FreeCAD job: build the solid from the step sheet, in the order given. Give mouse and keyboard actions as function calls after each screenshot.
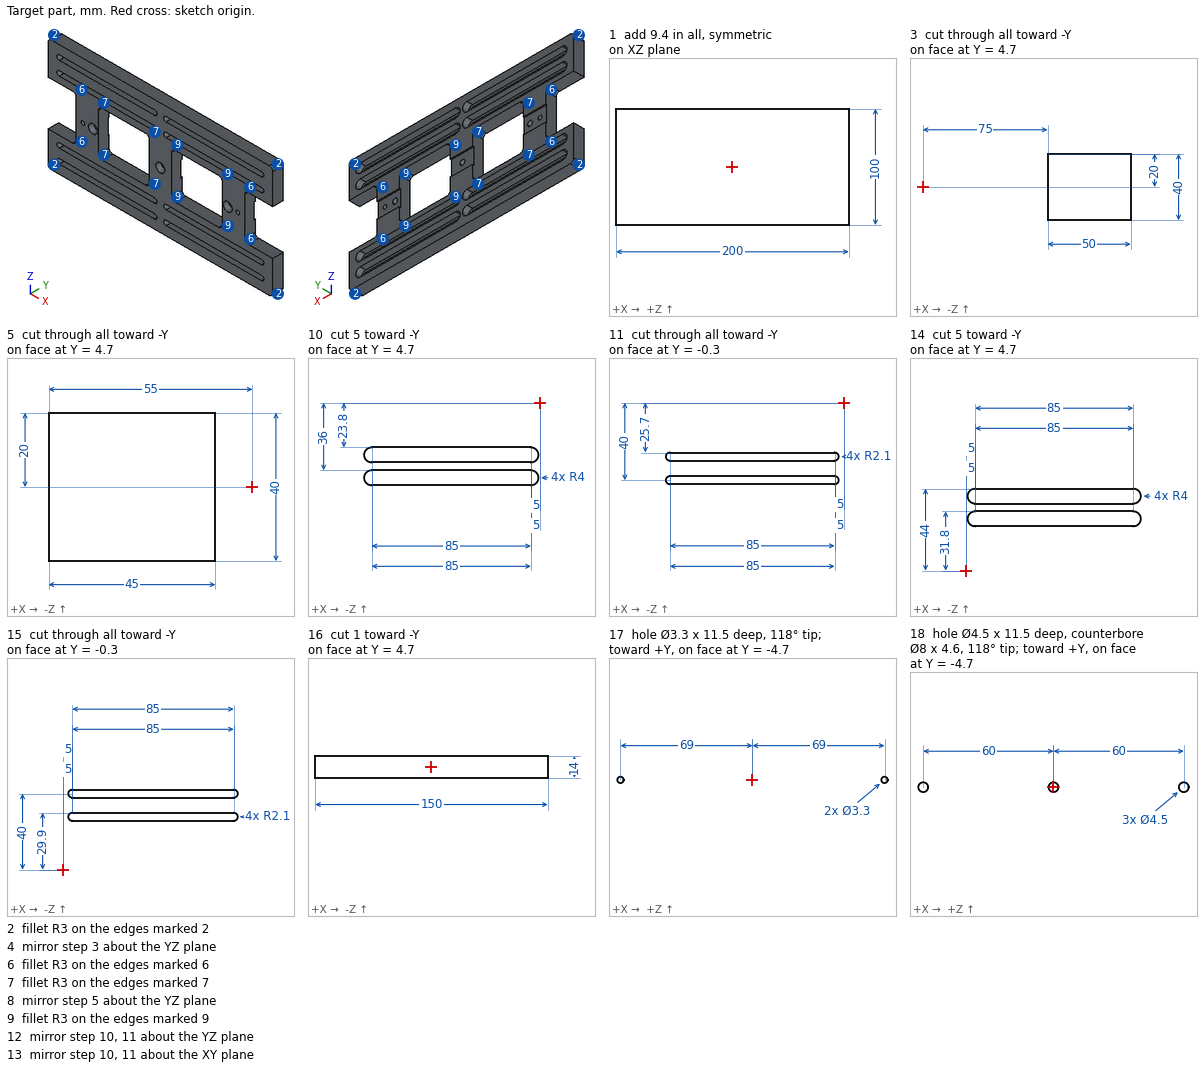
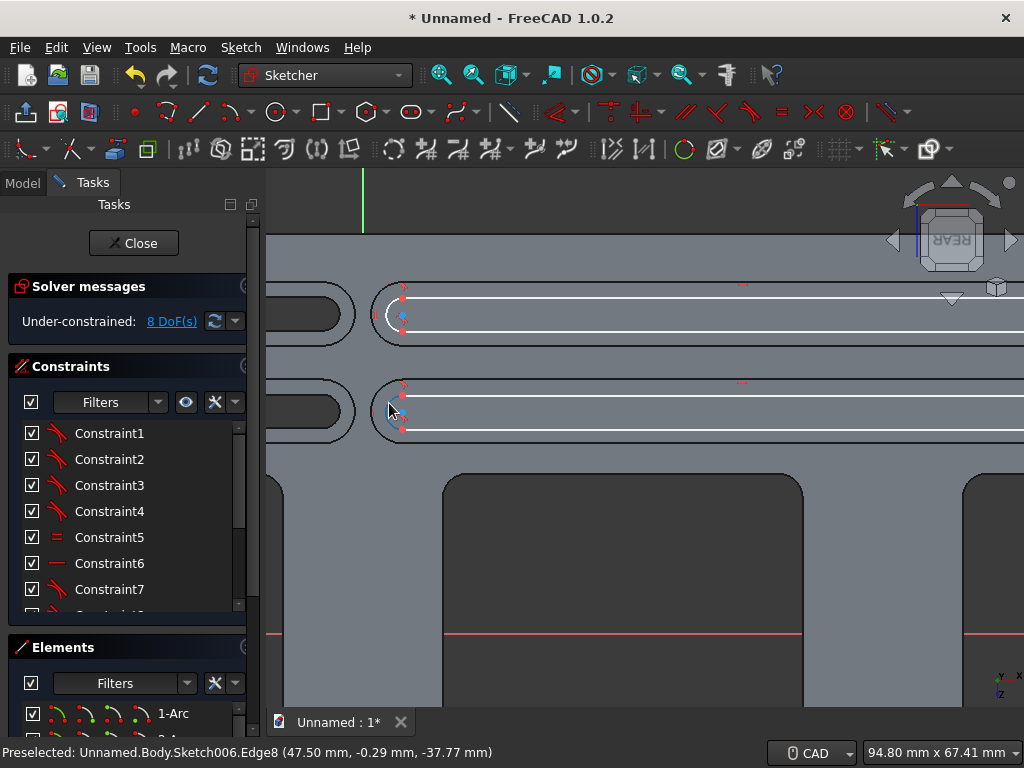
click(389, 403)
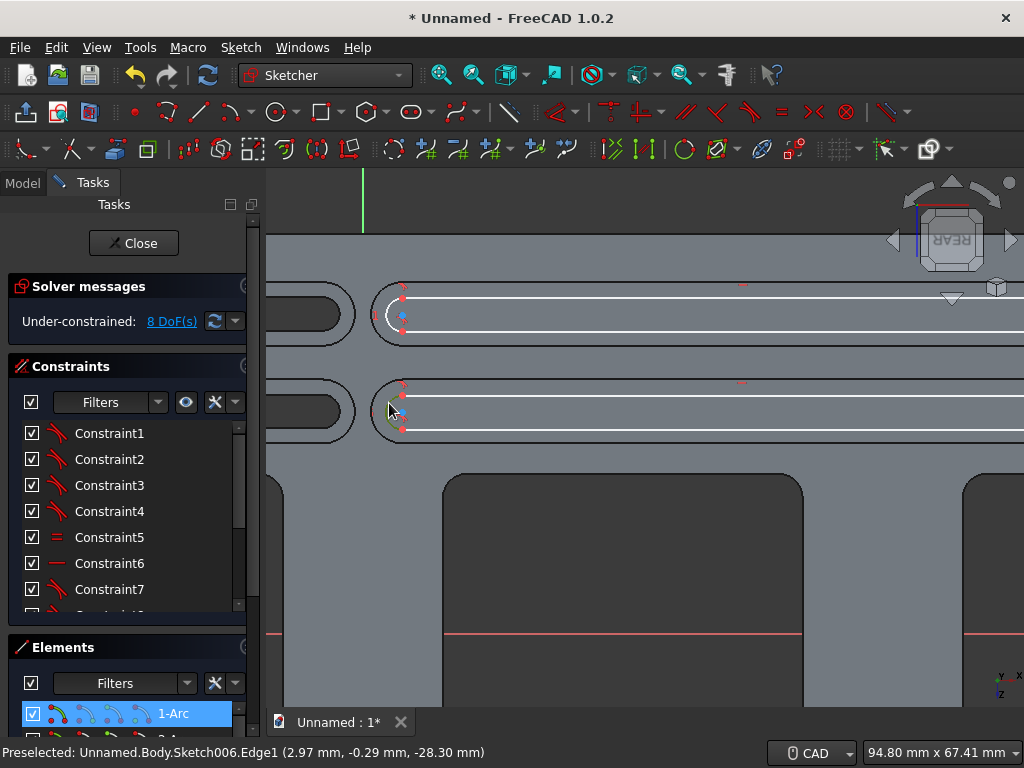
click(389, 305)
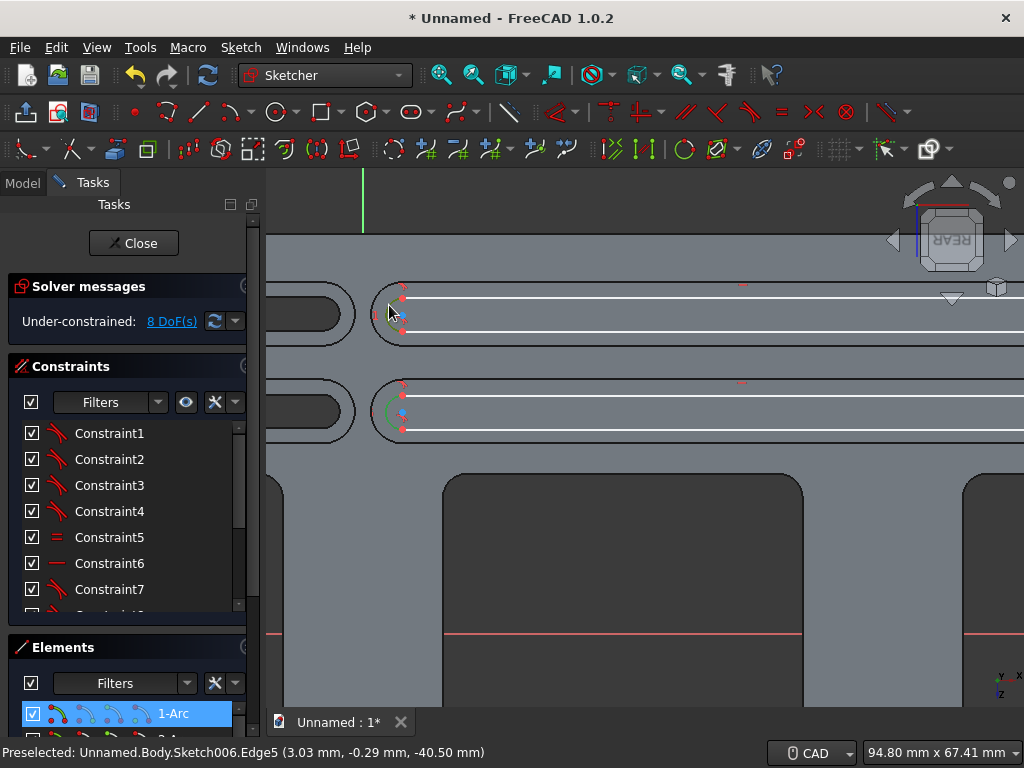
key(e)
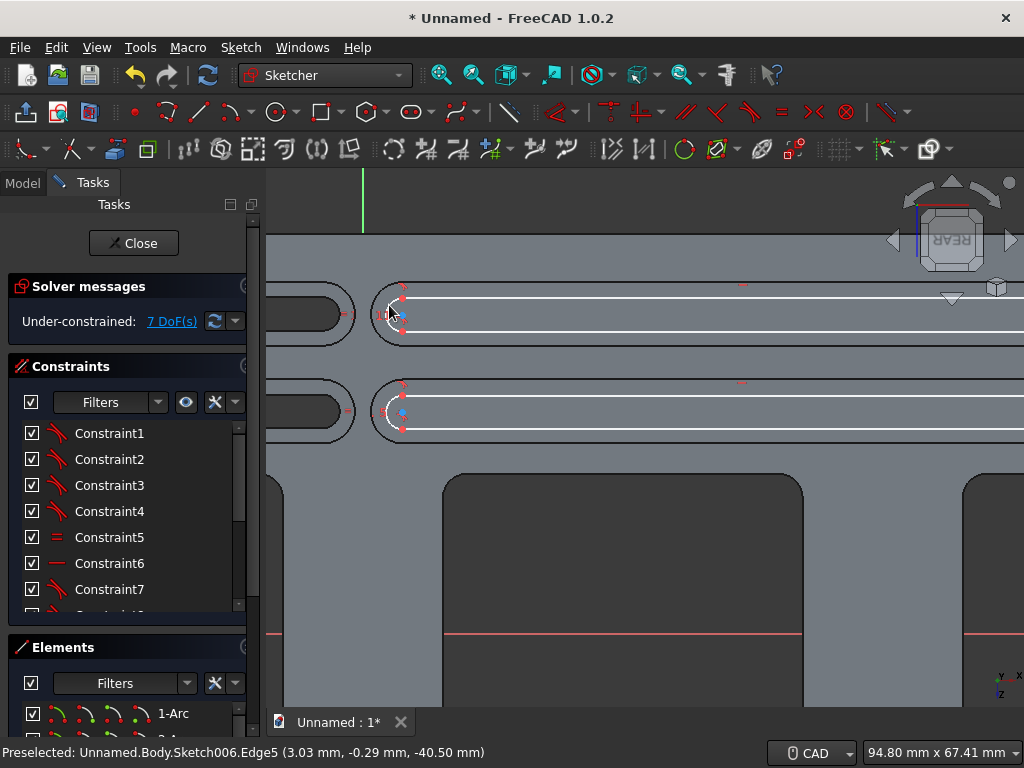
key(d)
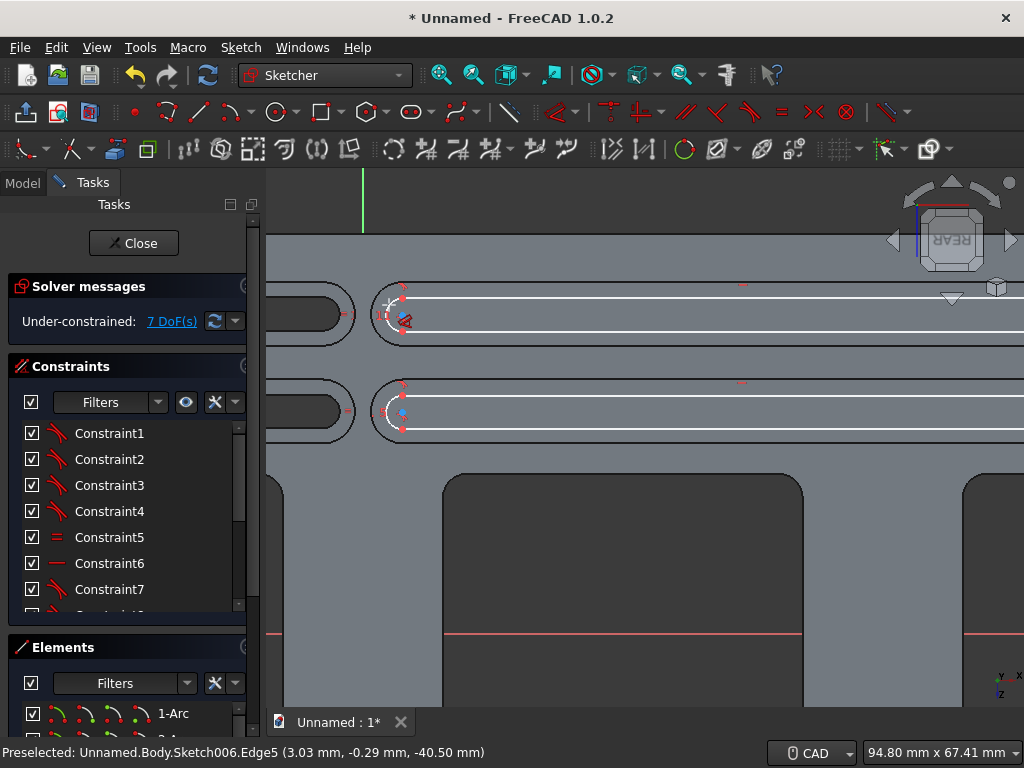
scroll(389, 403, up, 5)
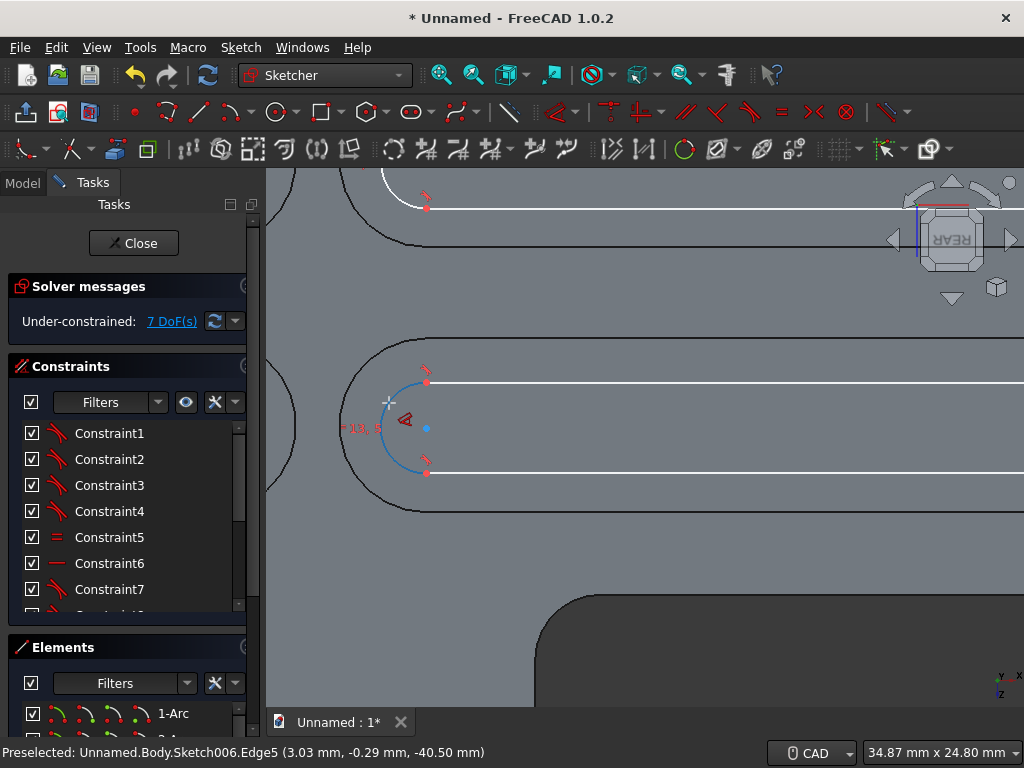
click(389, 401)
click(363, 382)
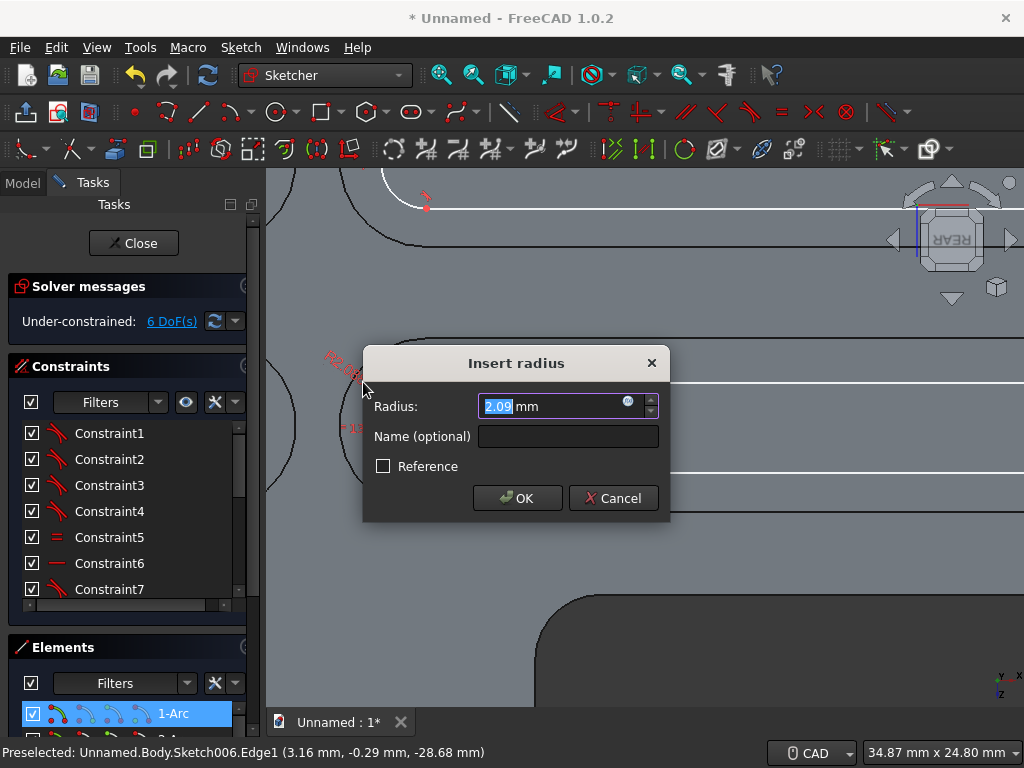
text(2.1)
key(Return)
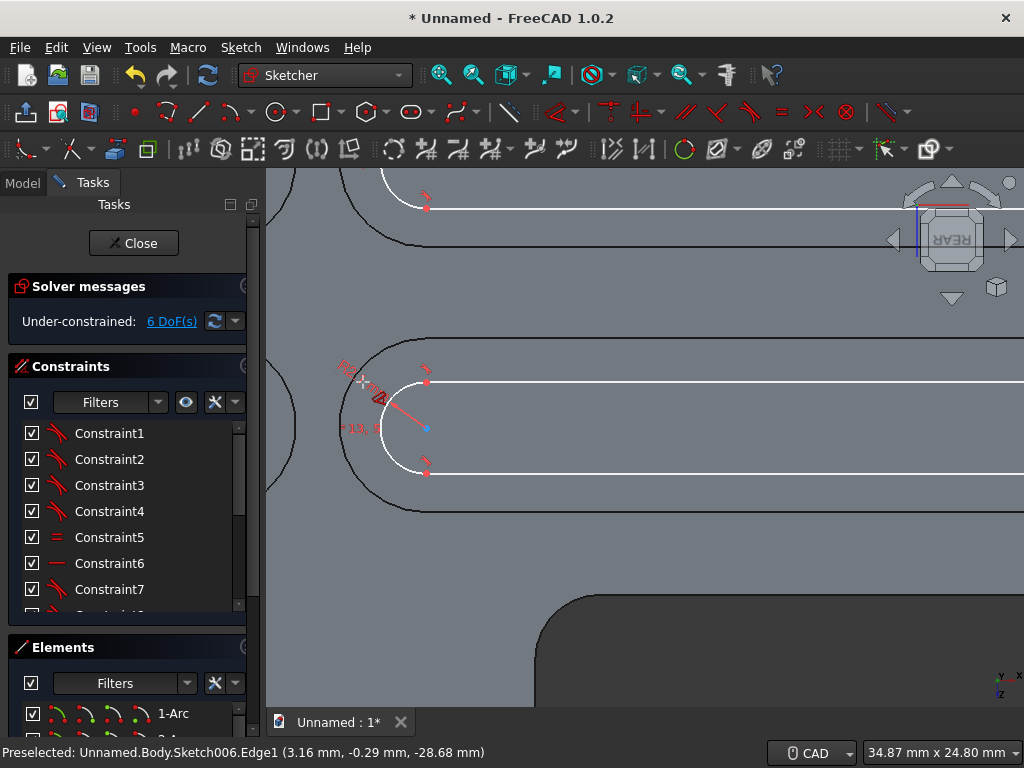
scroll(389, 403, down, 8)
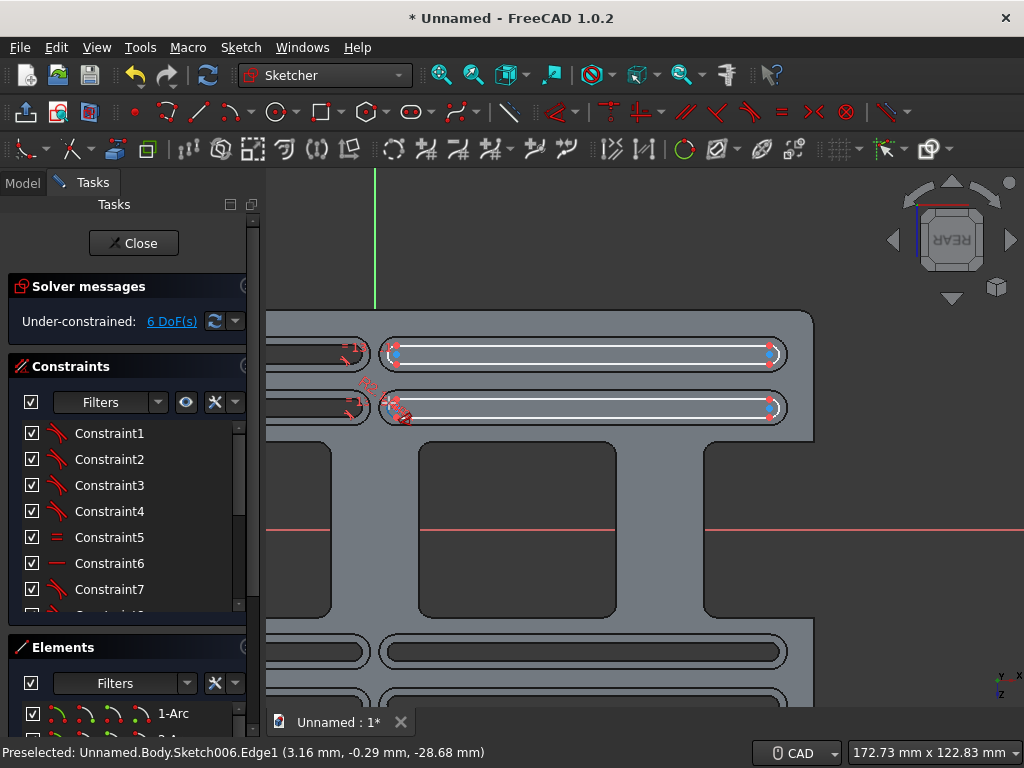
click(471, 399)
click(583, 433)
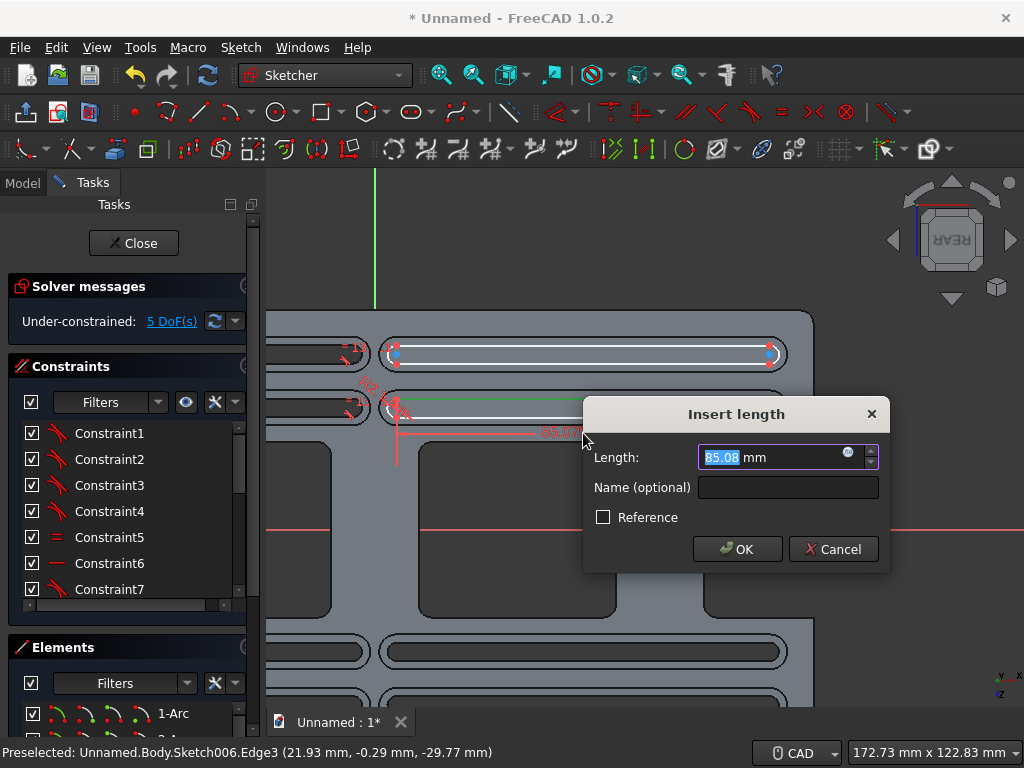
text(85)
key(Return)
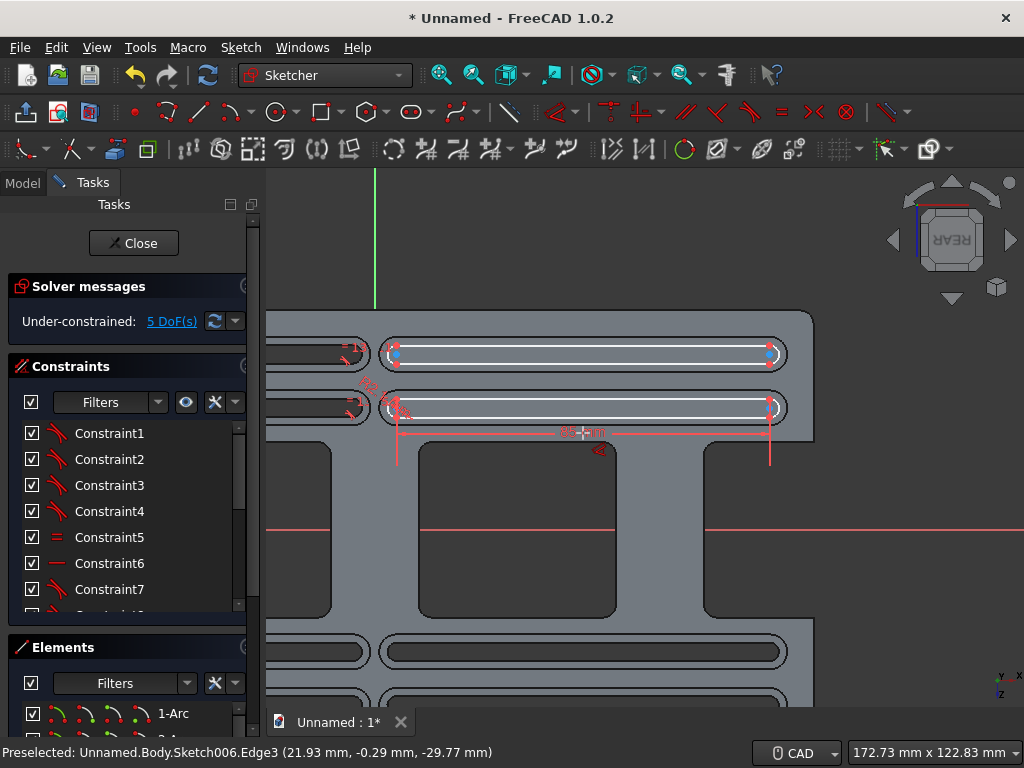
click(509, 346)
click(583, 312)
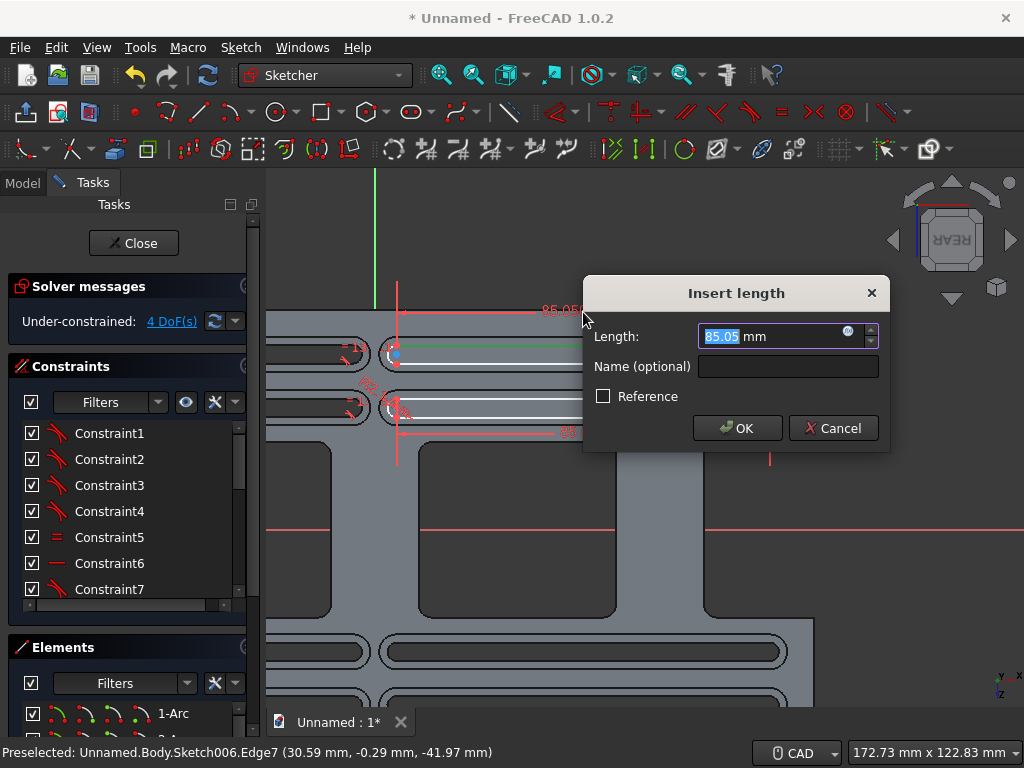
text(85)
key(Return)